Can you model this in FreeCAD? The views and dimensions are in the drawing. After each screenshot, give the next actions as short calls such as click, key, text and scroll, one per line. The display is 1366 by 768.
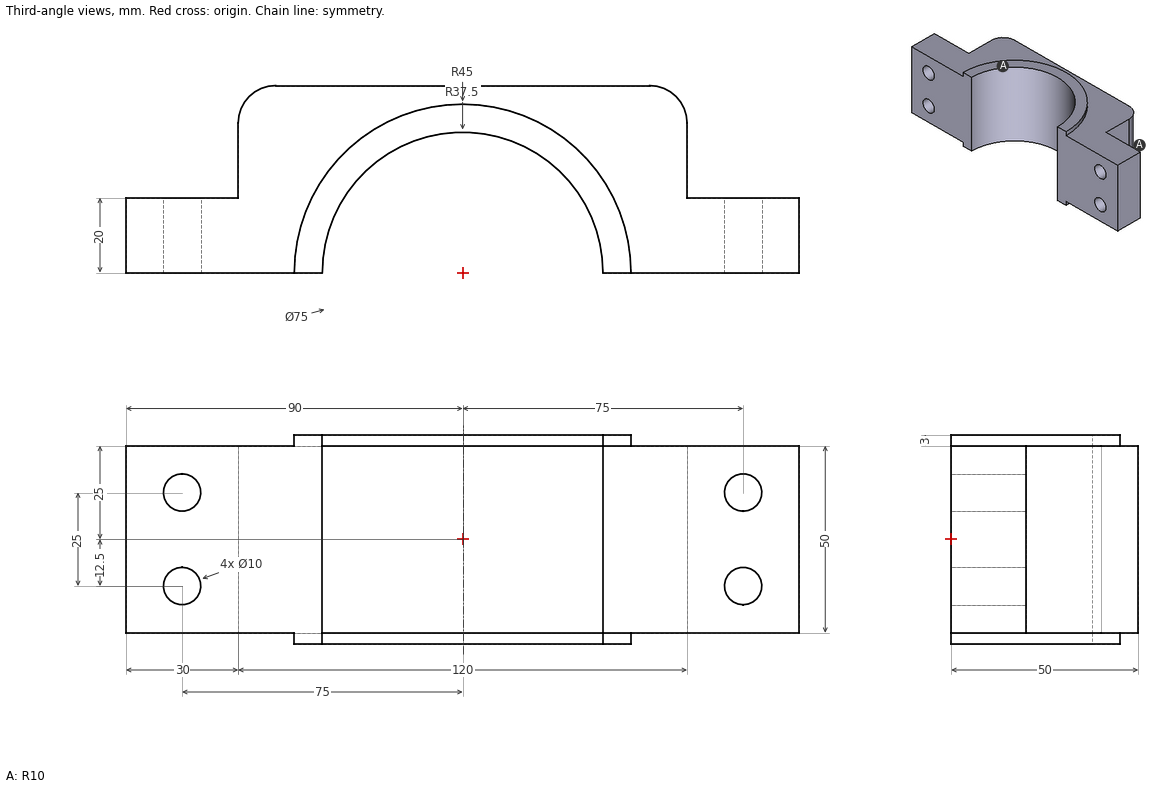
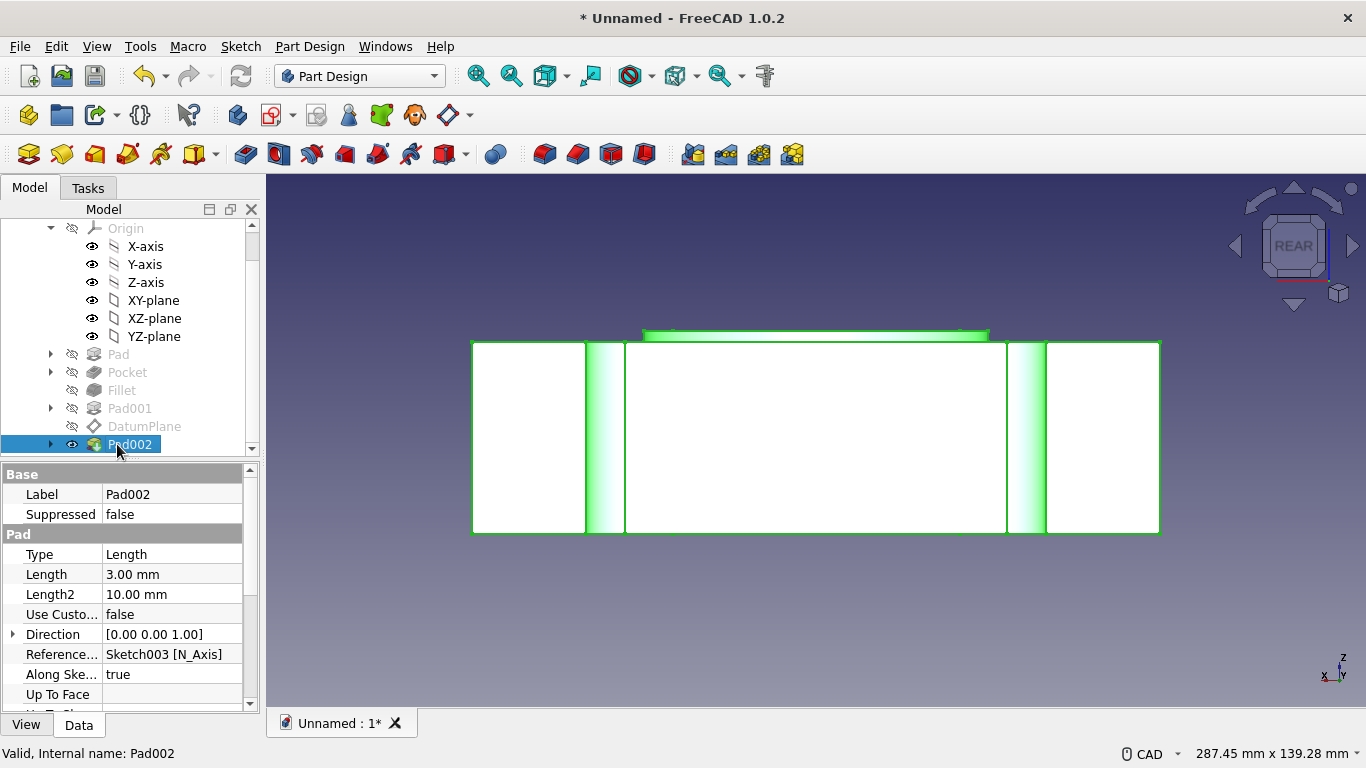
click(693, 154)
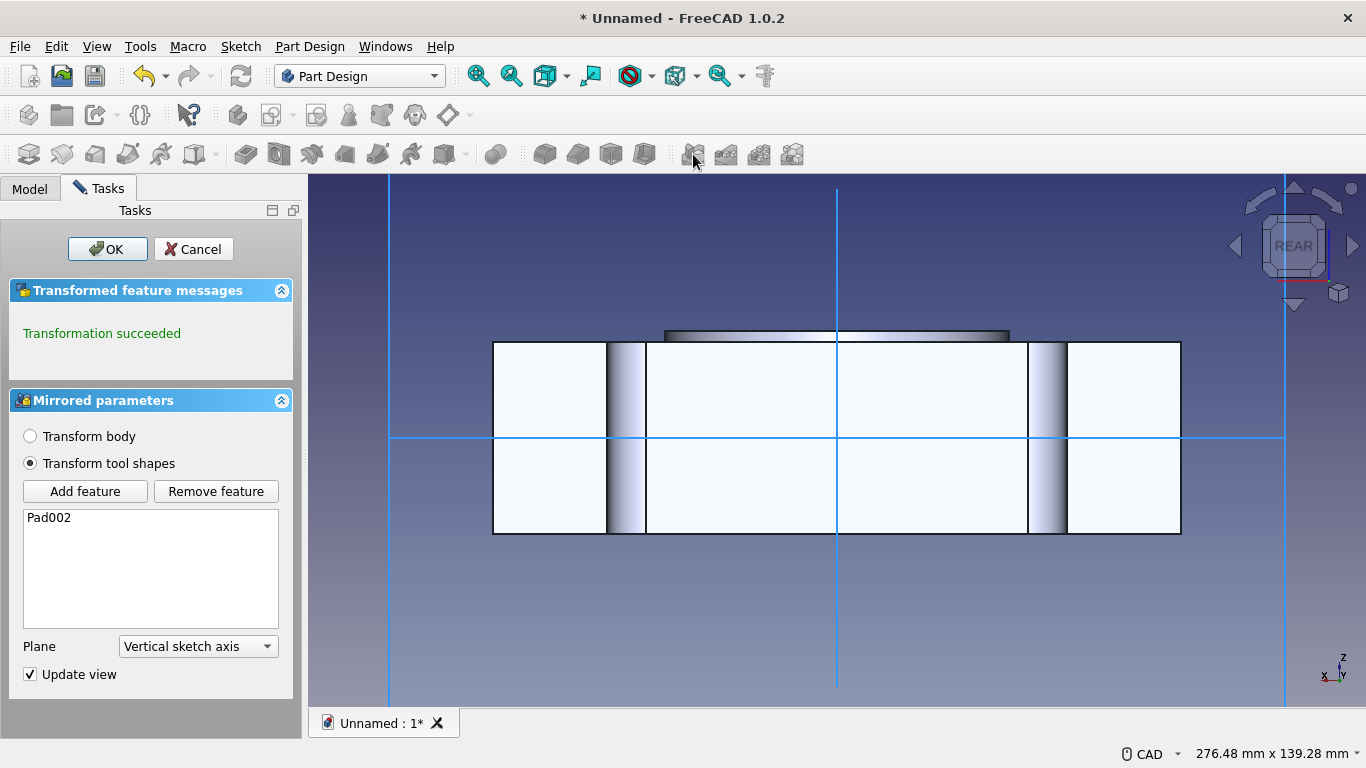
click(199, 646)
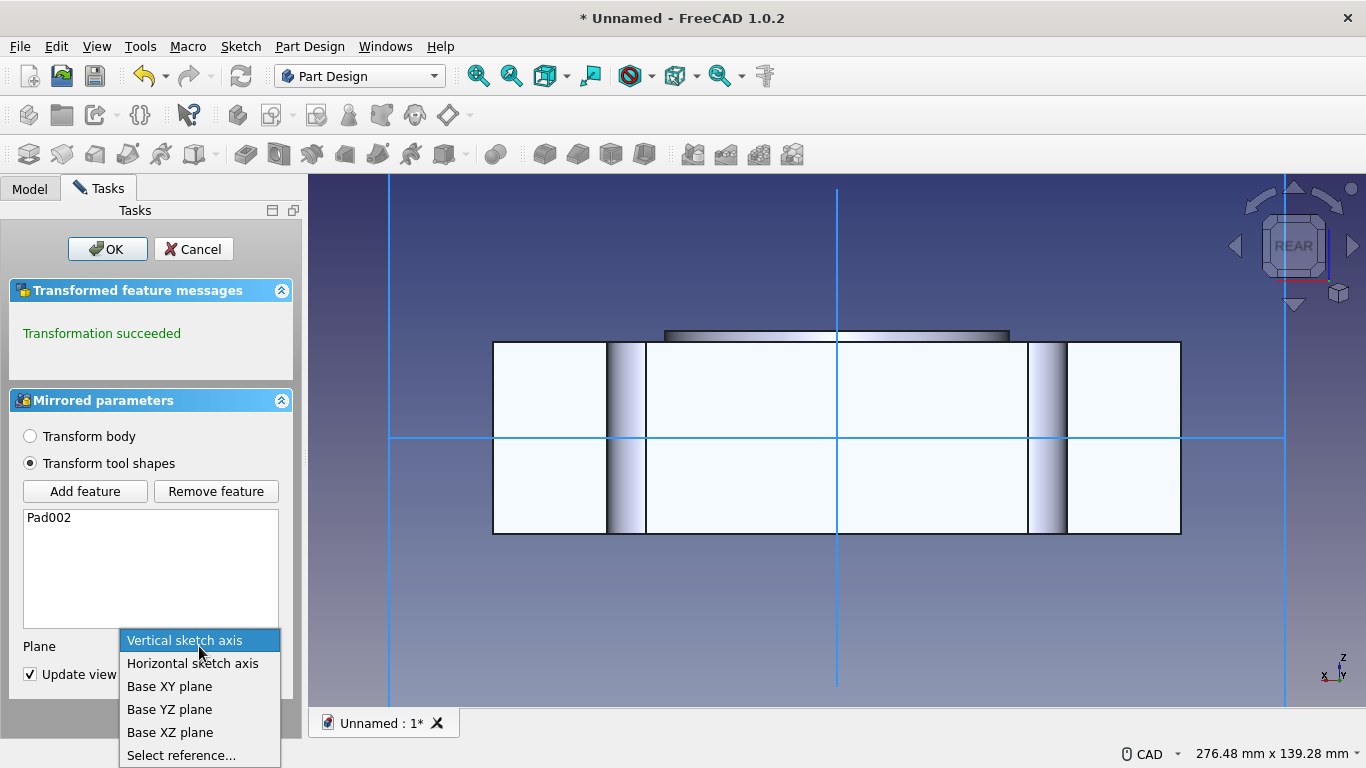
click(198, 686)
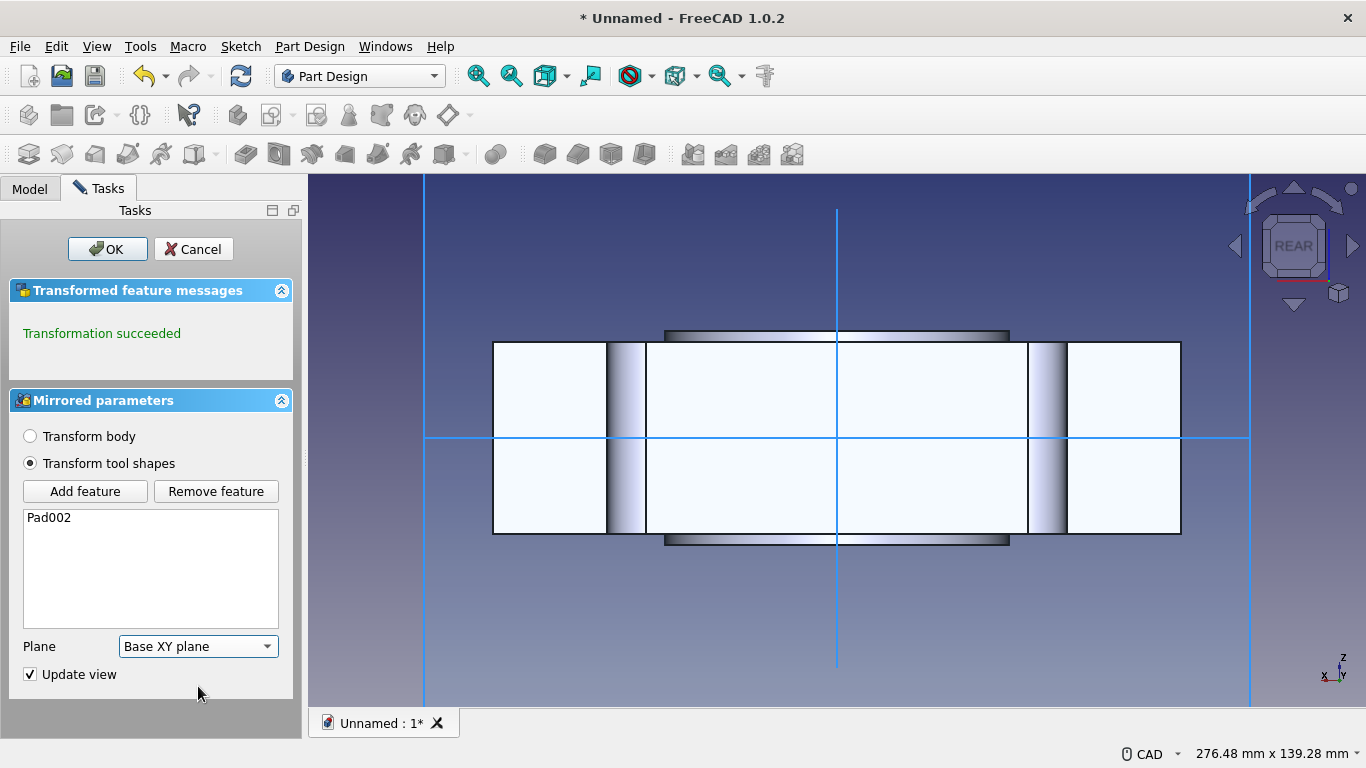
click(108, 249)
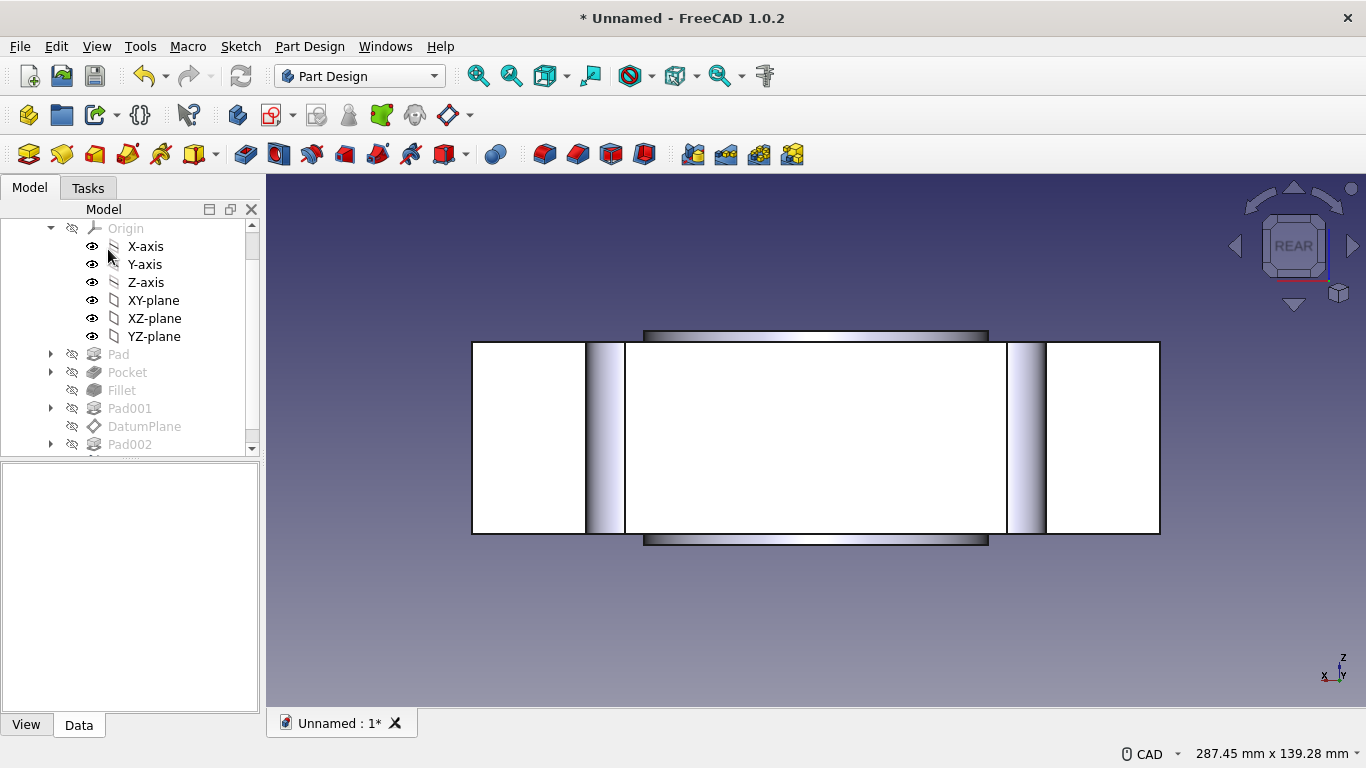
click(1103, 410)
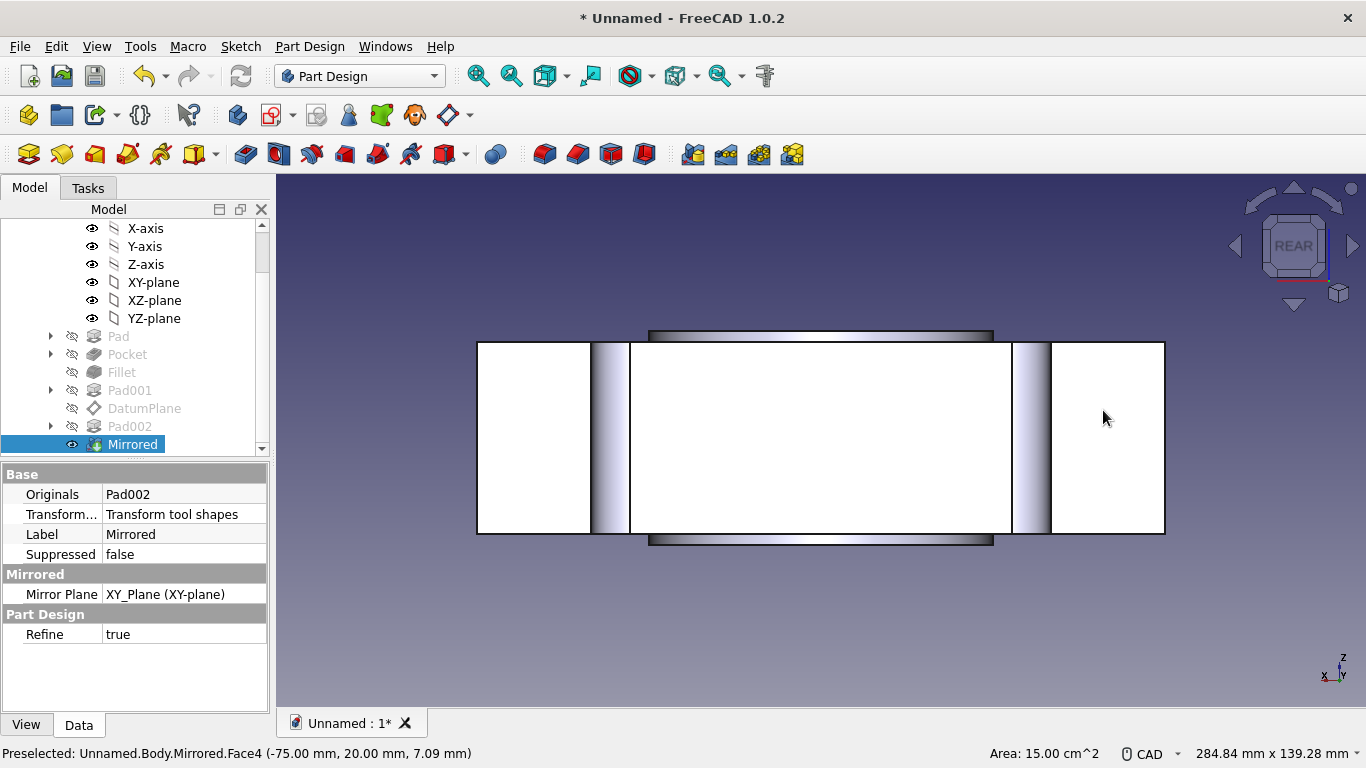
click(270, 116)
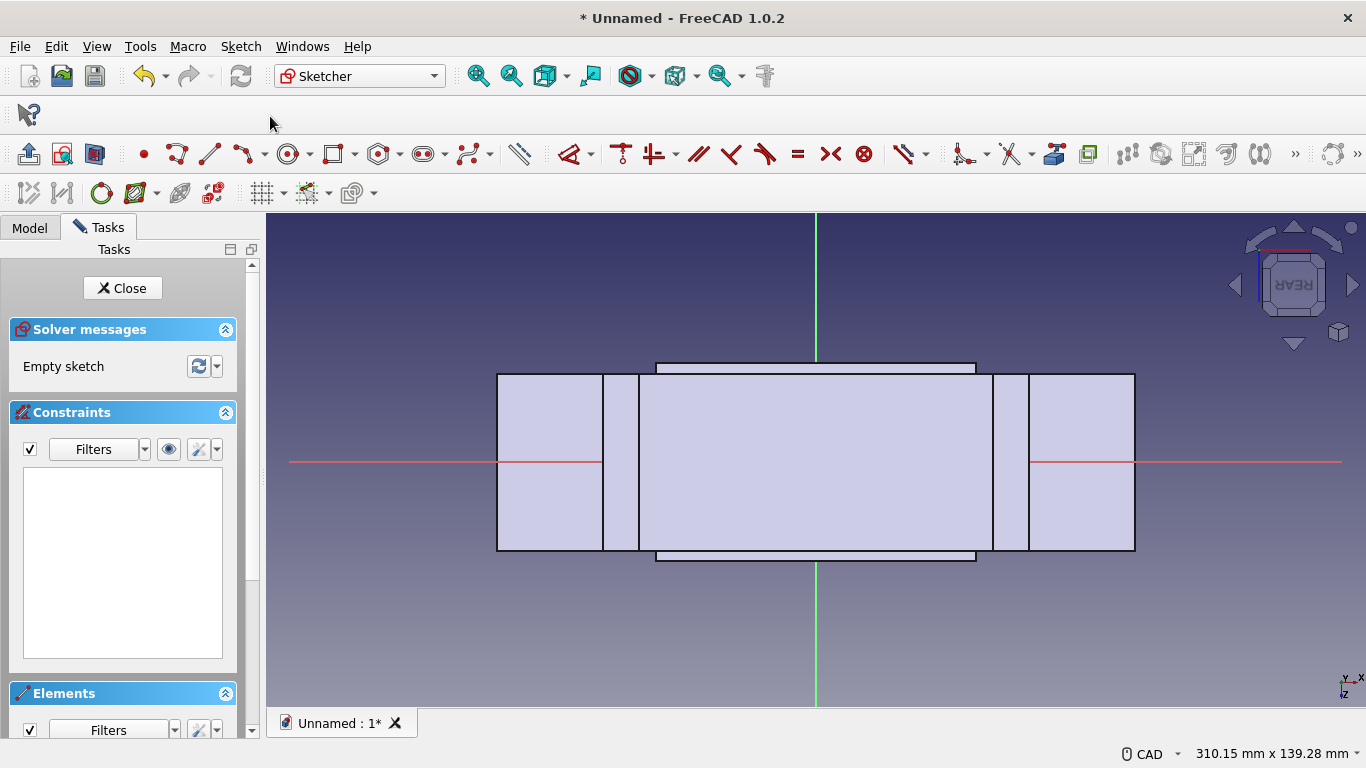
key(g)
key(c)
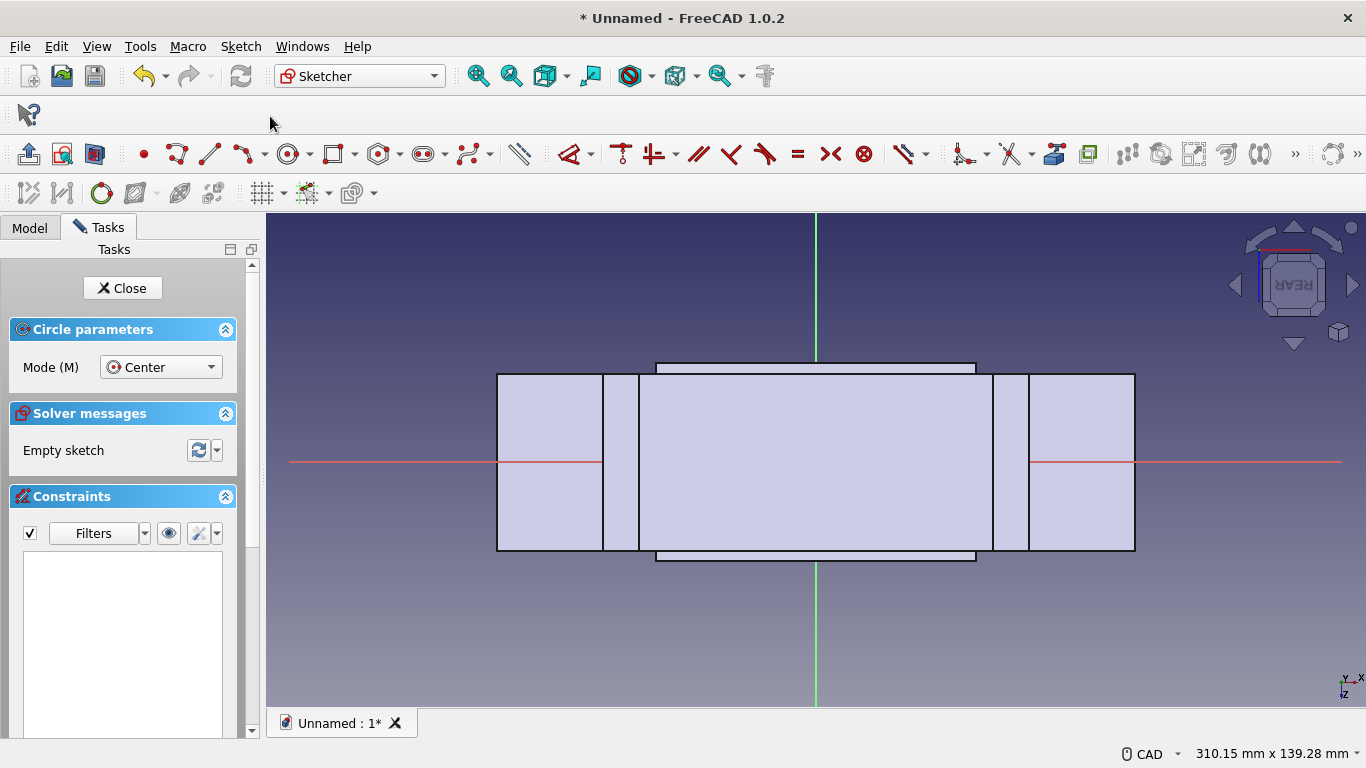
scroll(550, 418, up, 2)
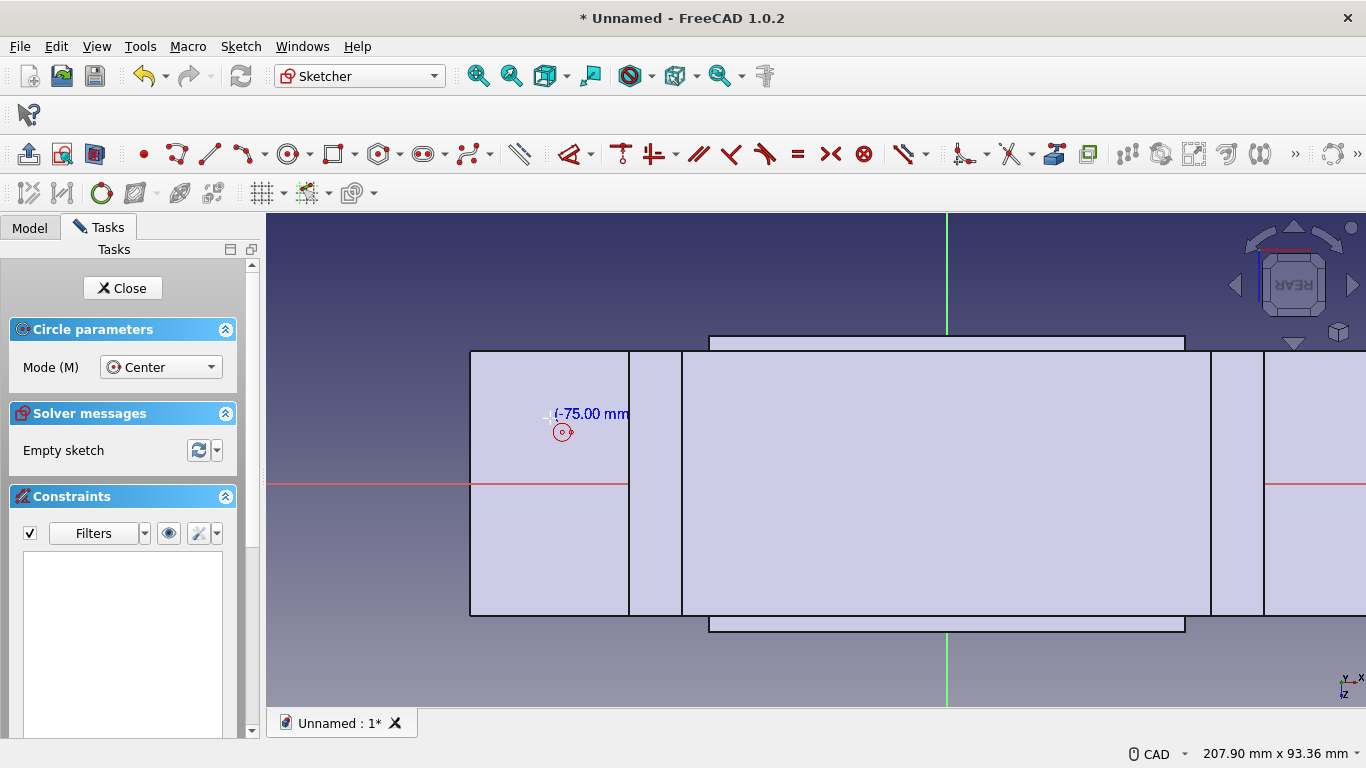
click(550, 418)
click(569, 399)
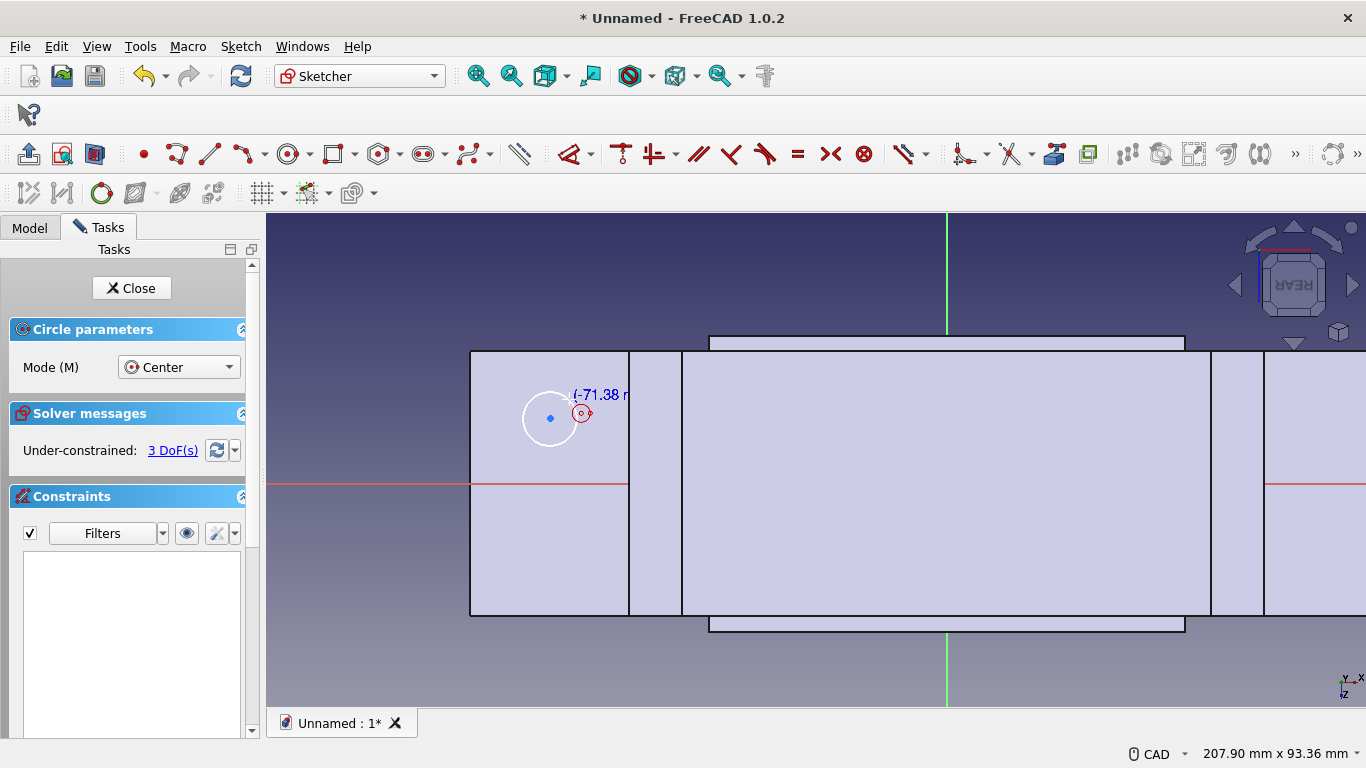
click(550, 550)
click(569, 531)